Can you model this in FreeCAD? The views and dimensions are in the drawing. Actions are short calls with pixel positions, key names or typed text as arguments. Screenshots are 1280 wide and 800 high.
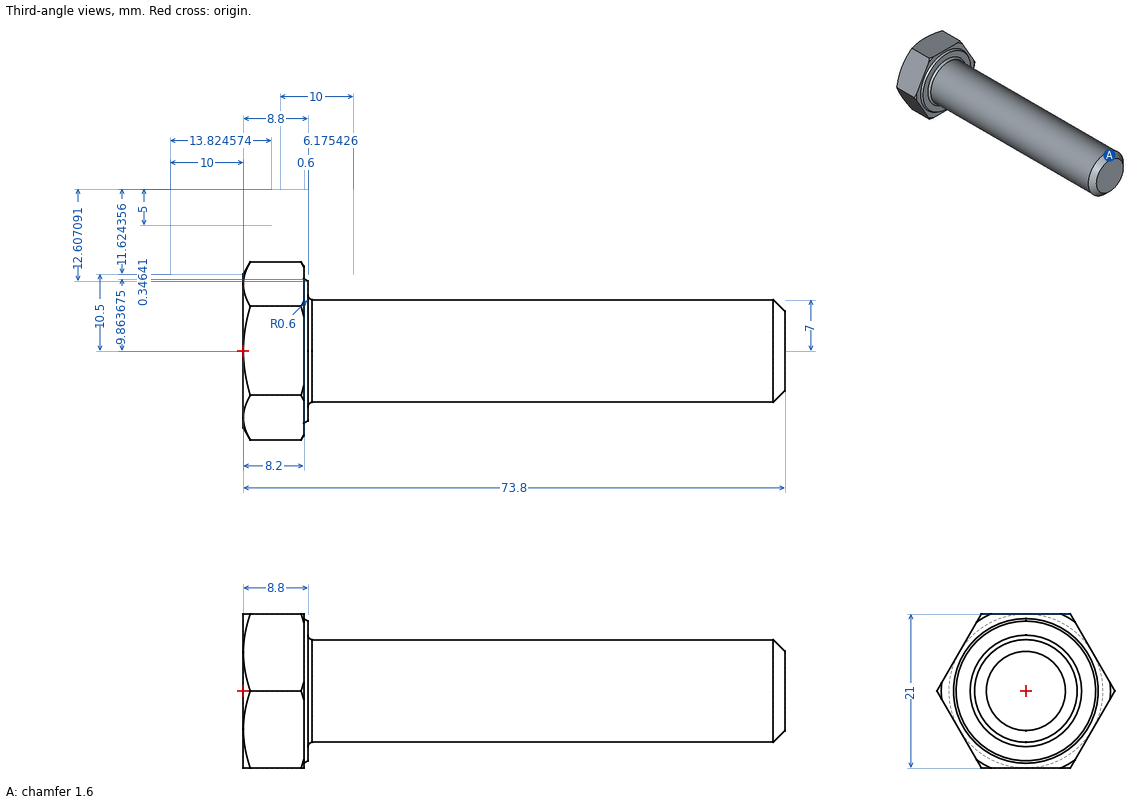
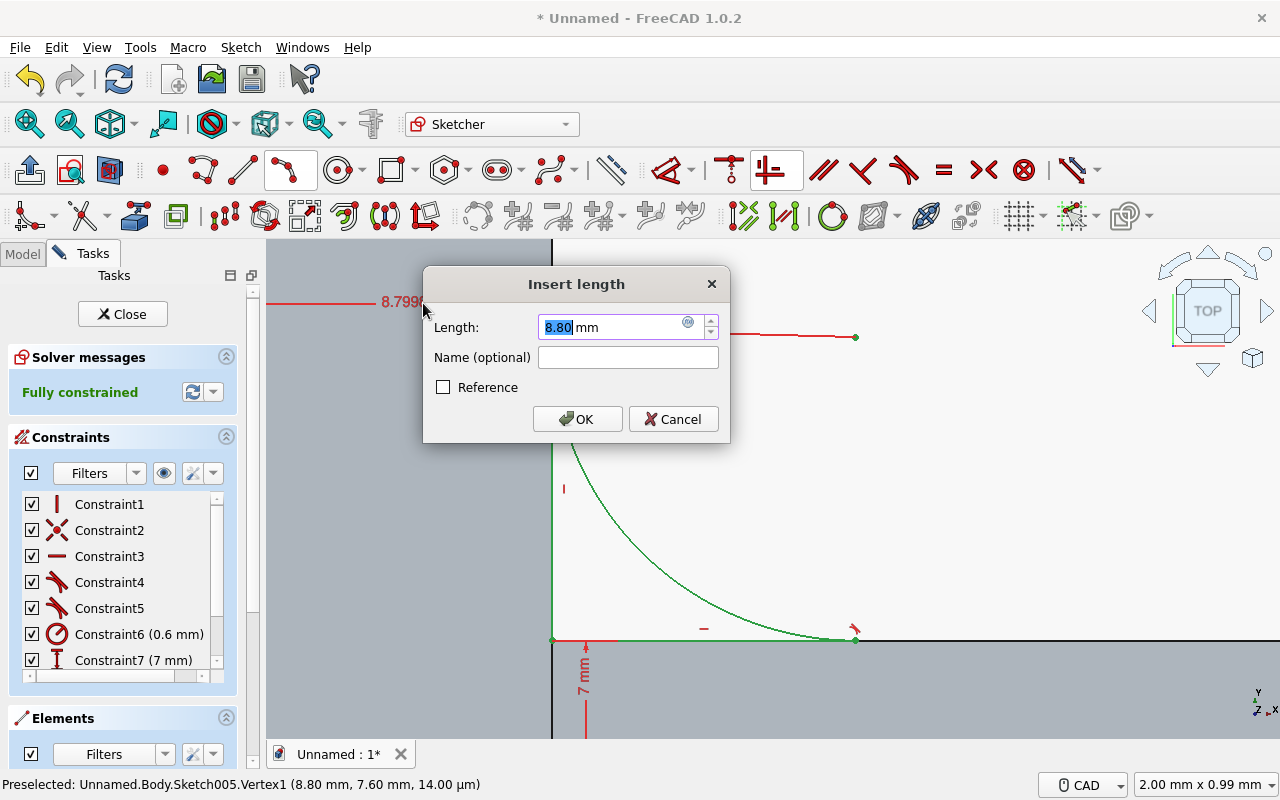
text(8.8)
key(Return)
key(Escape)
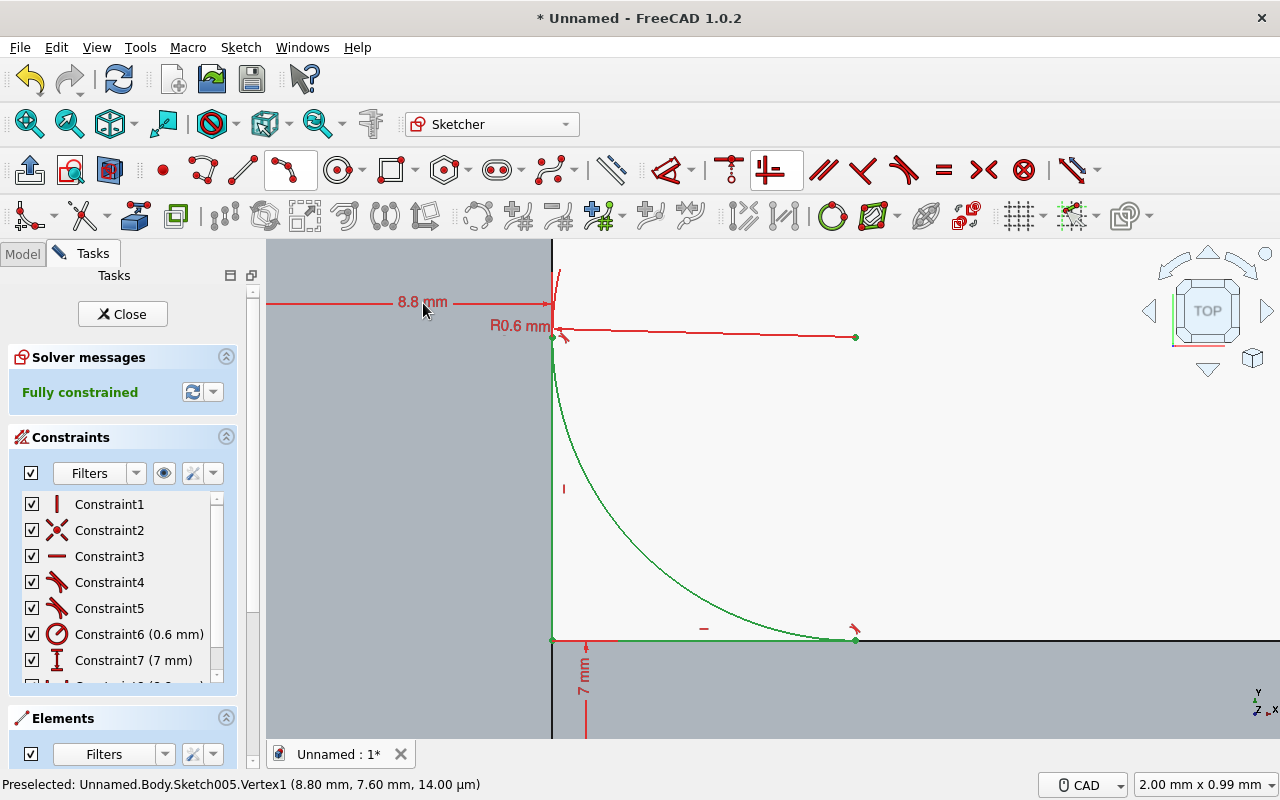
click(123, 314)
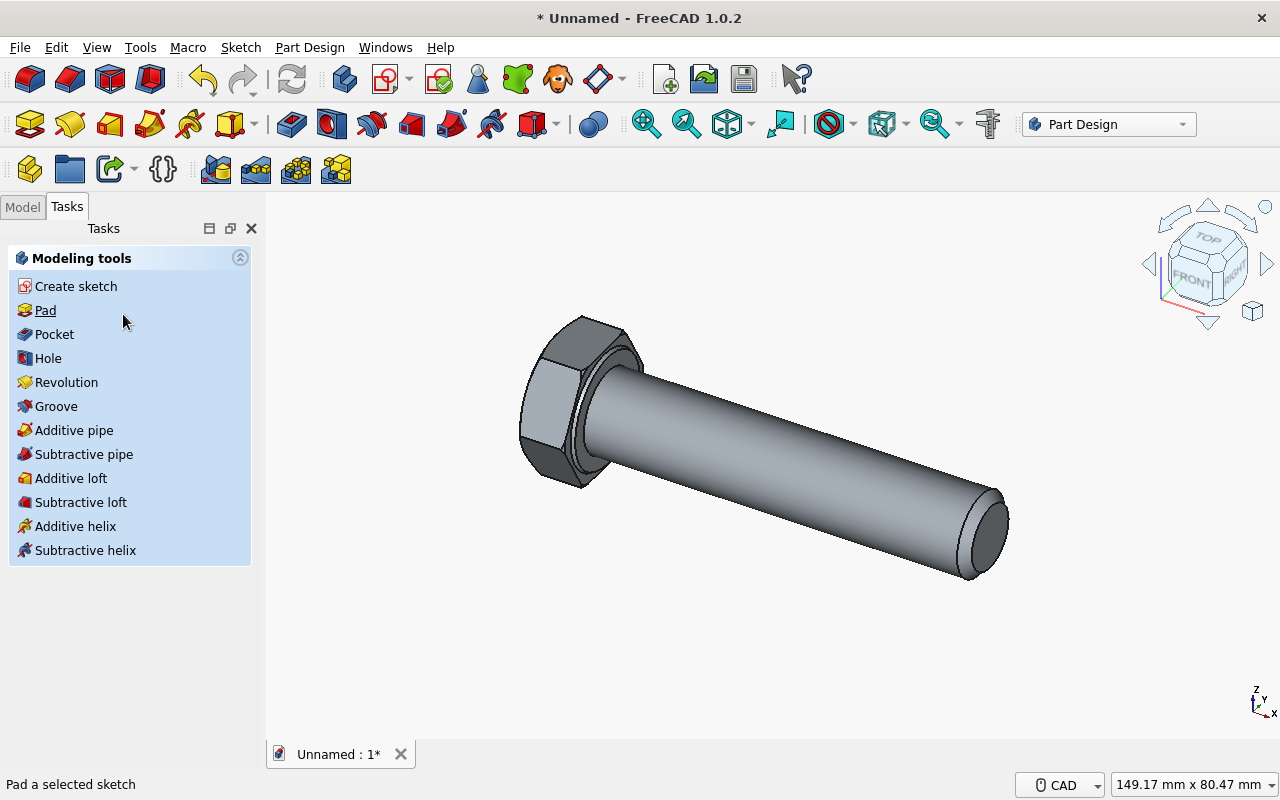
click(70, 124)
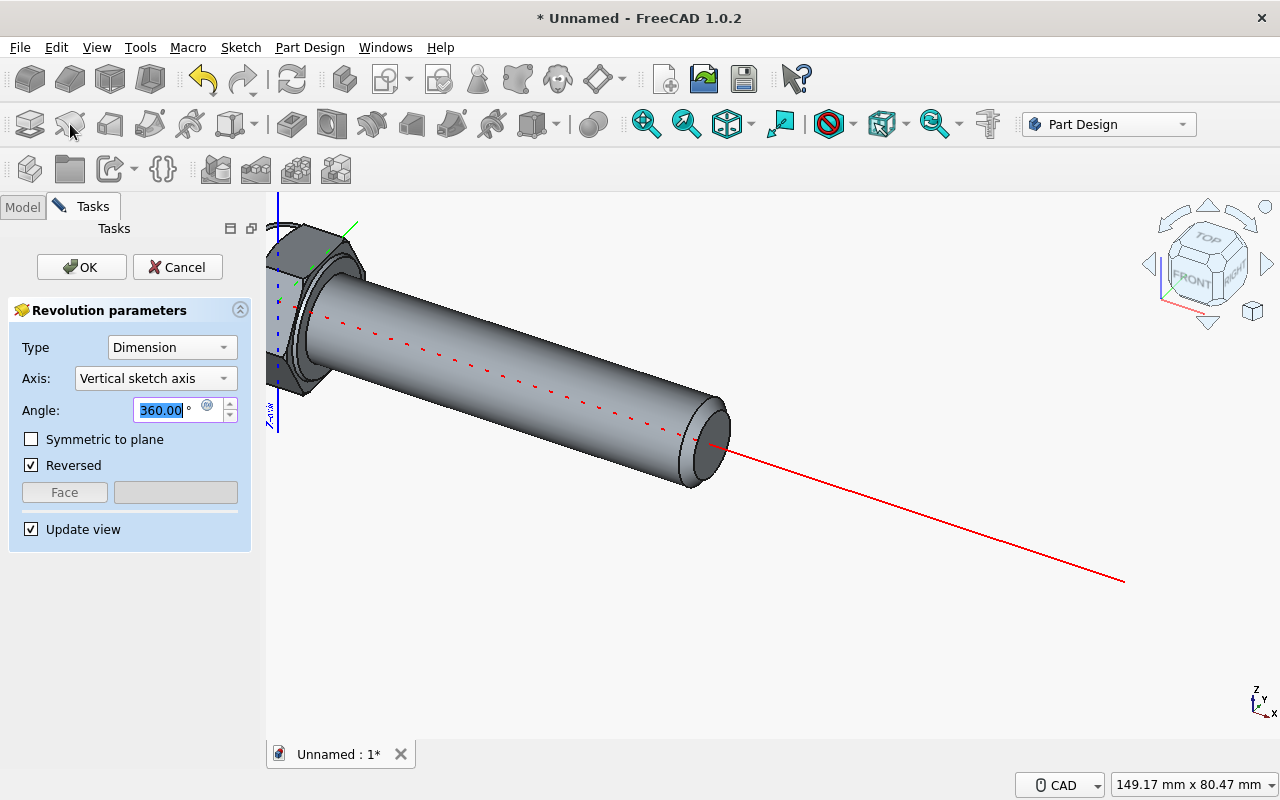
click(156, 378)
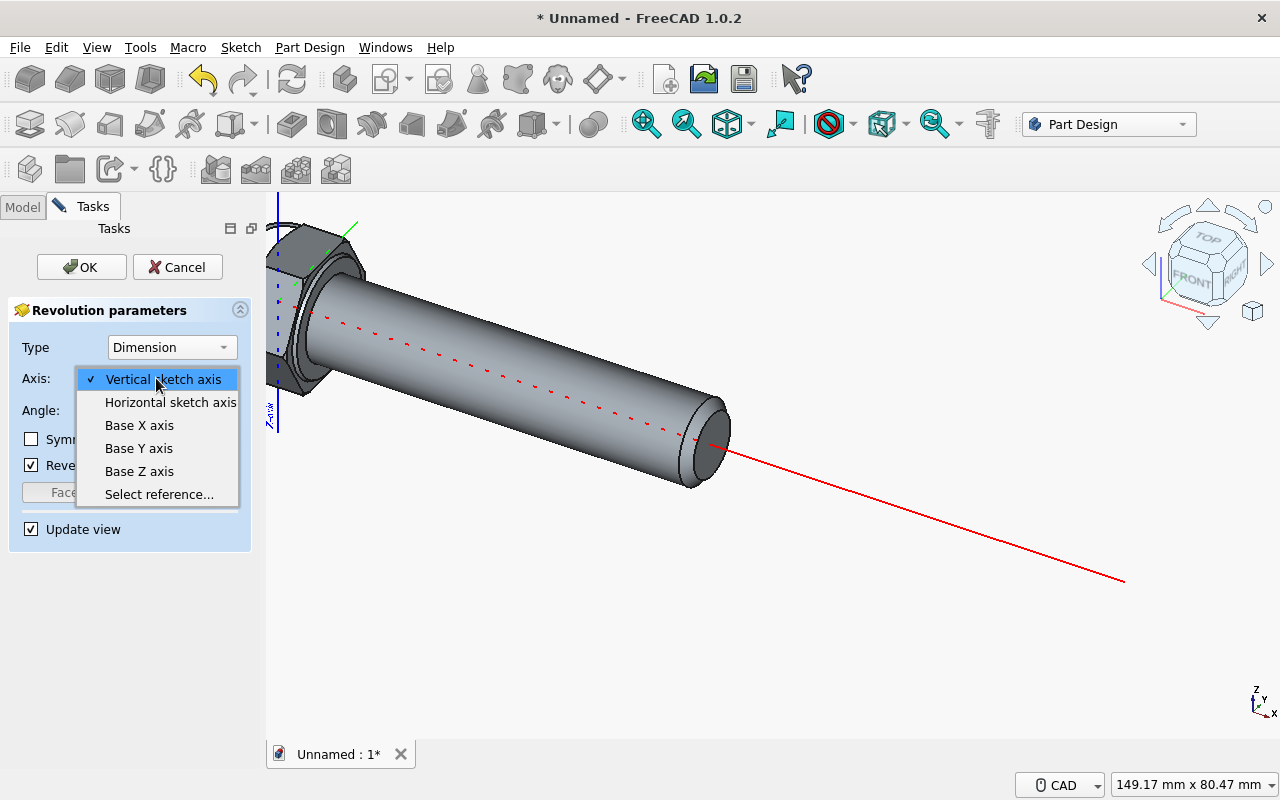
click(156, 402)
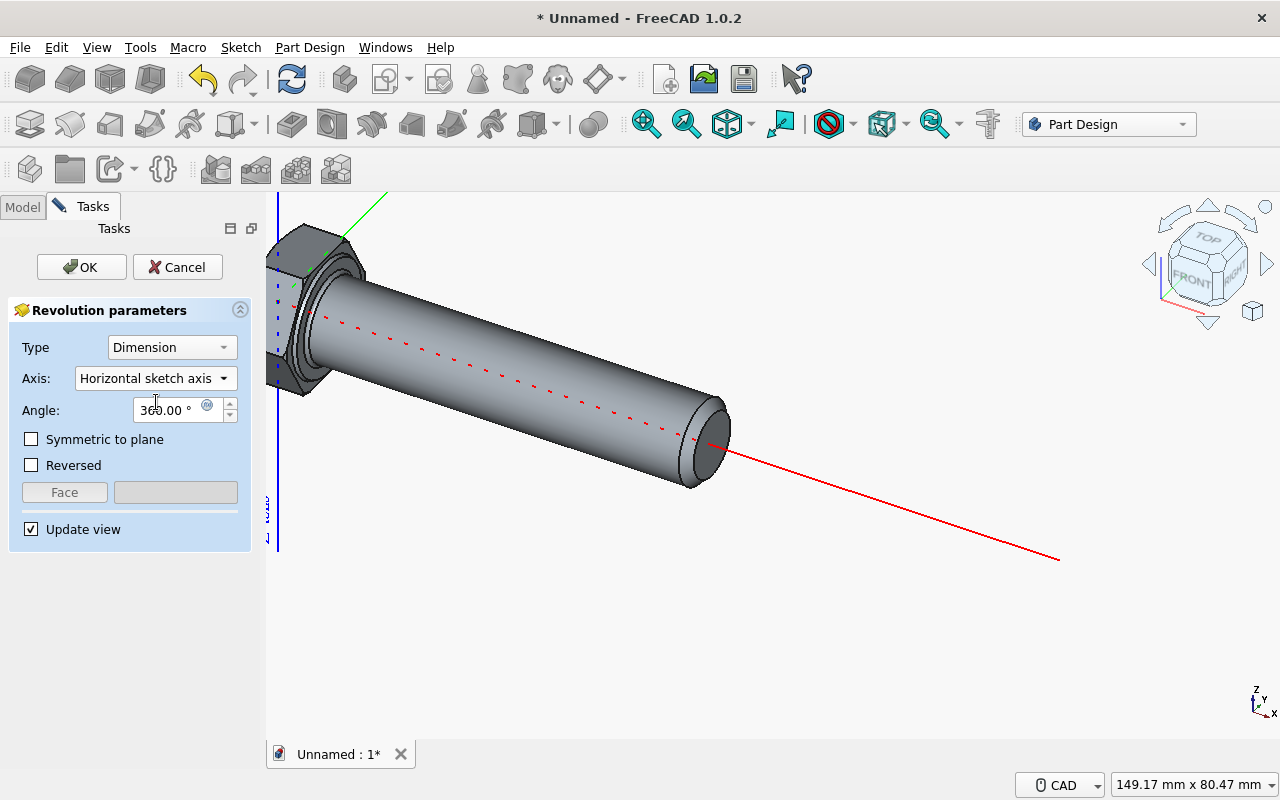
click(82, 267)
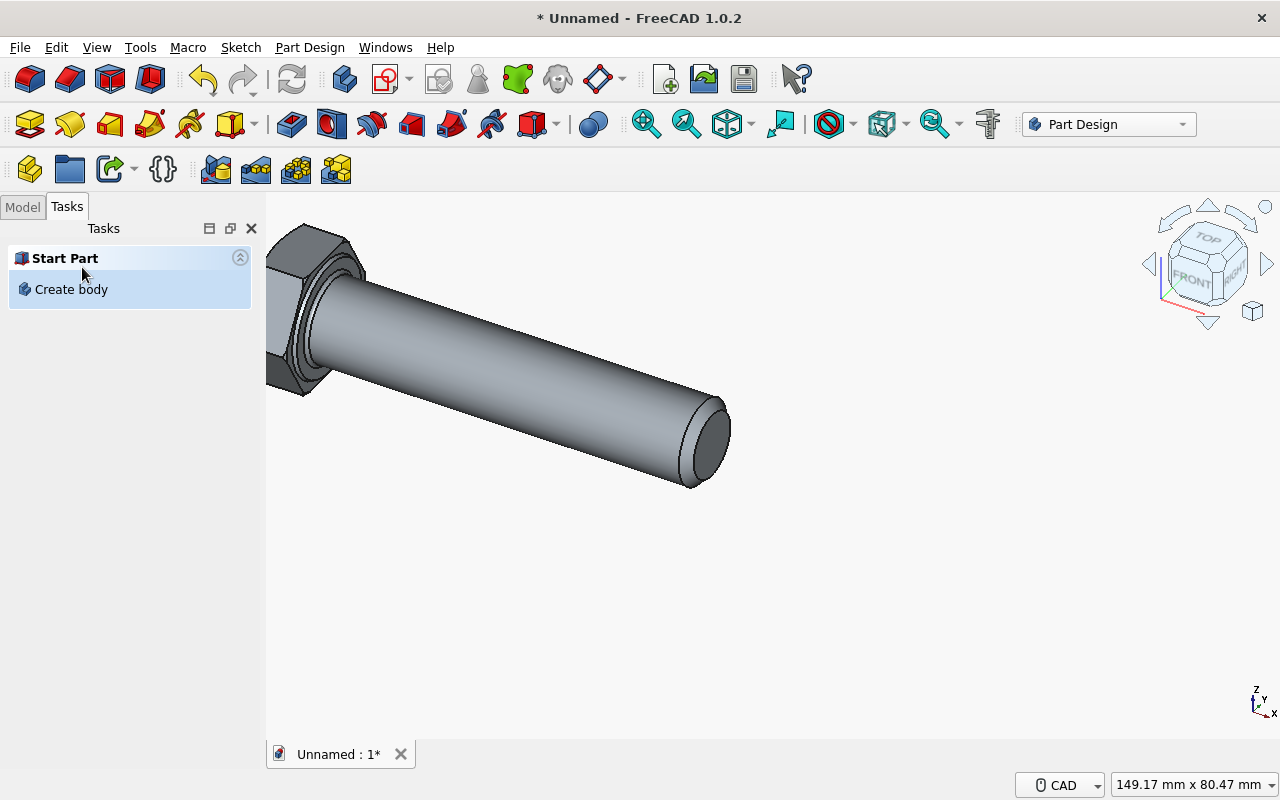
key(0)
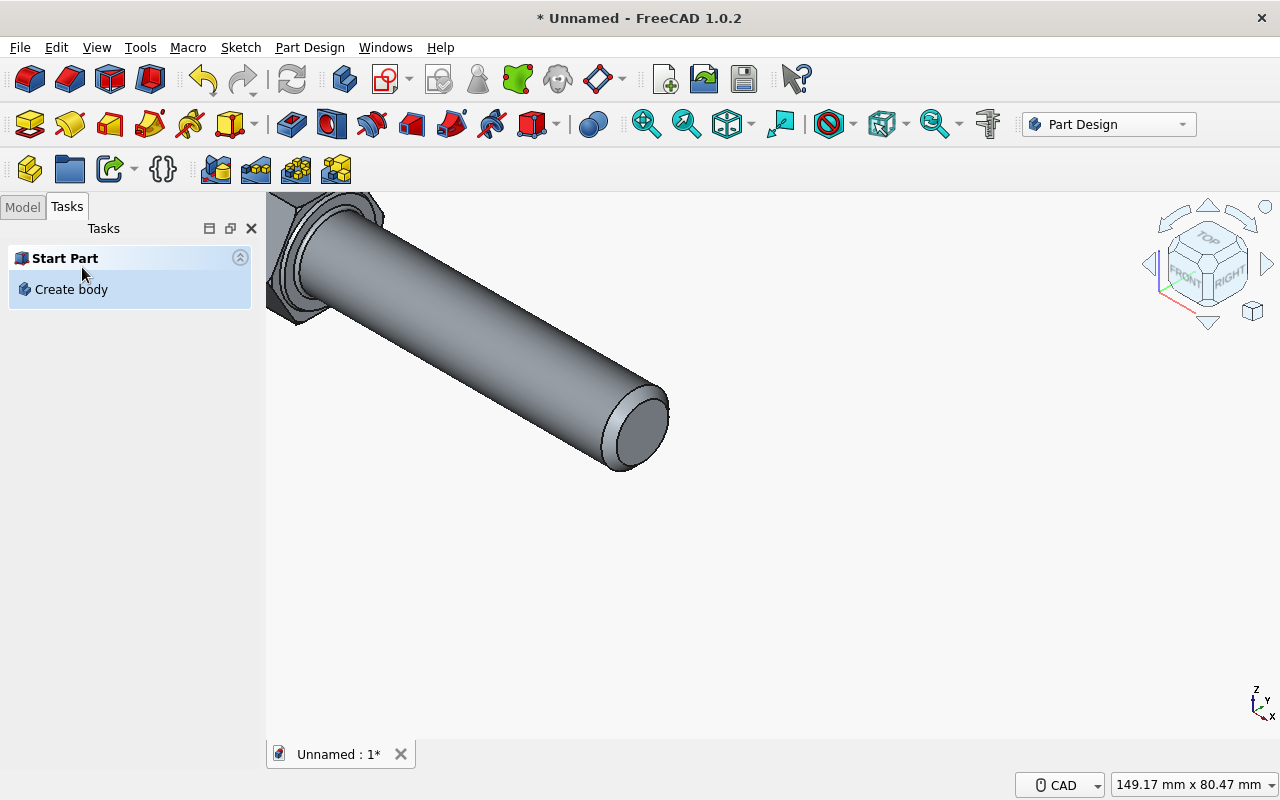
click(648, 124)